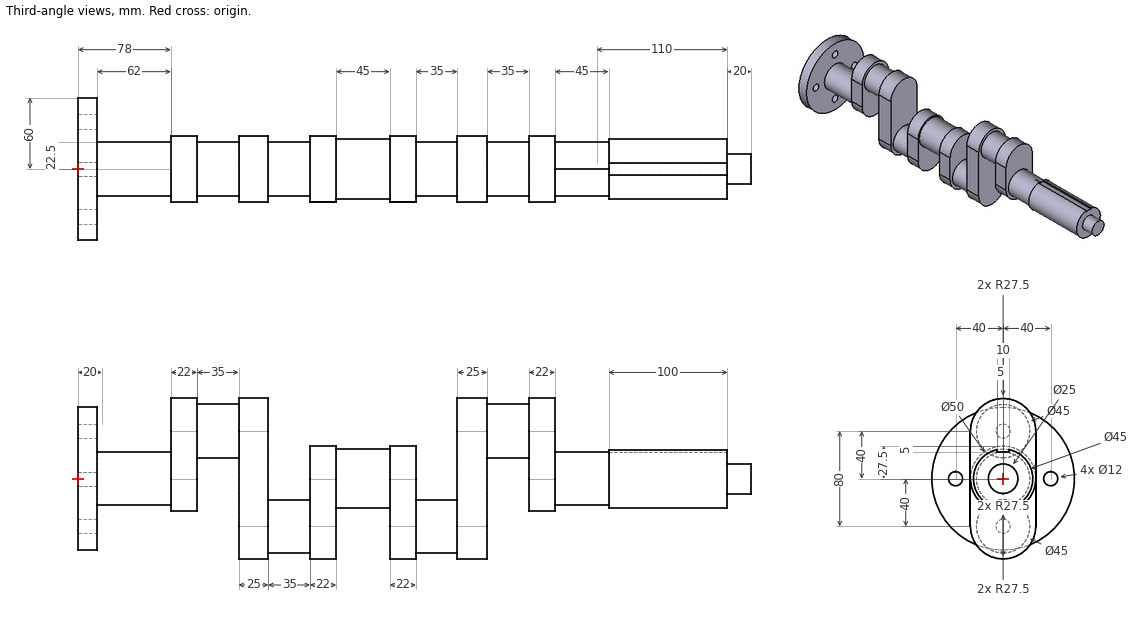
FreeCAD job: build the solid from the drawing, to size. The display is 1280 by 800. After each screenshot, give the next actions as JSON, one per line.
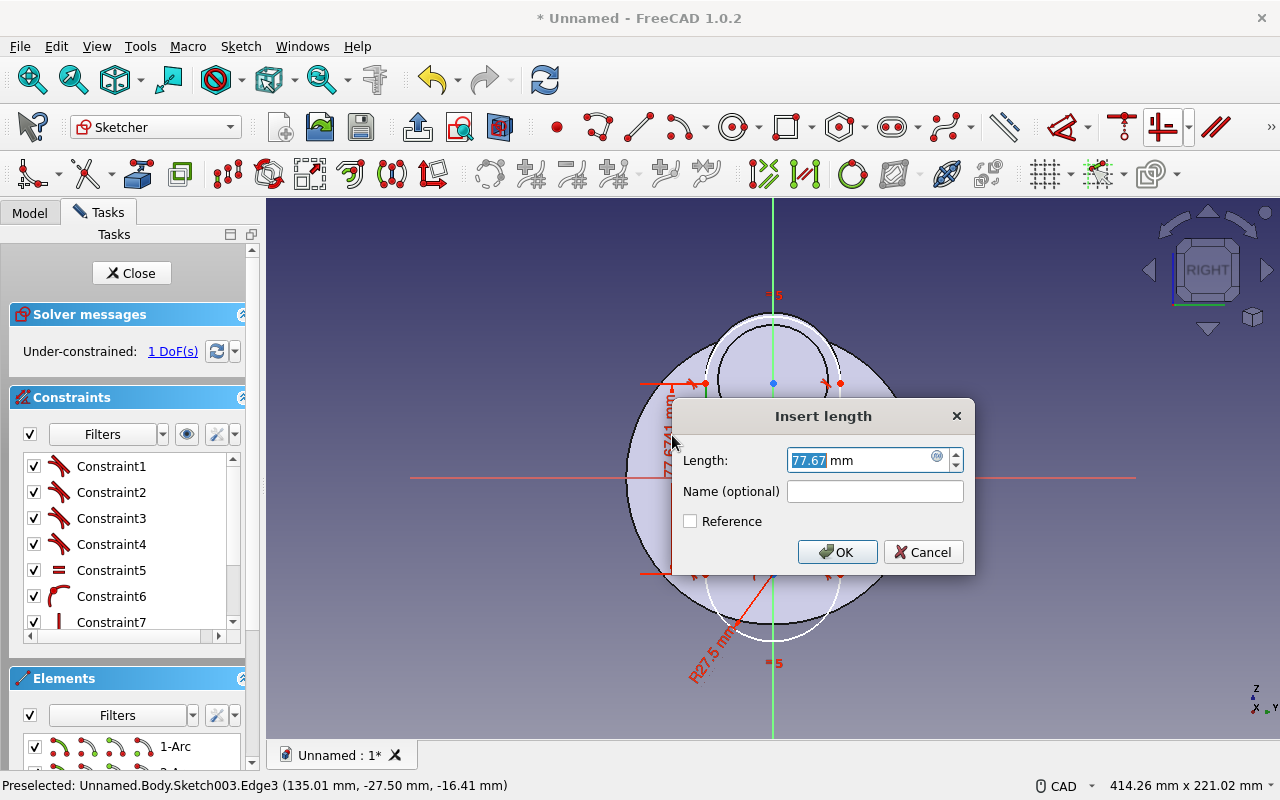
{"action": "type", "text": "80"}
{"action": "key", "text": "Return"}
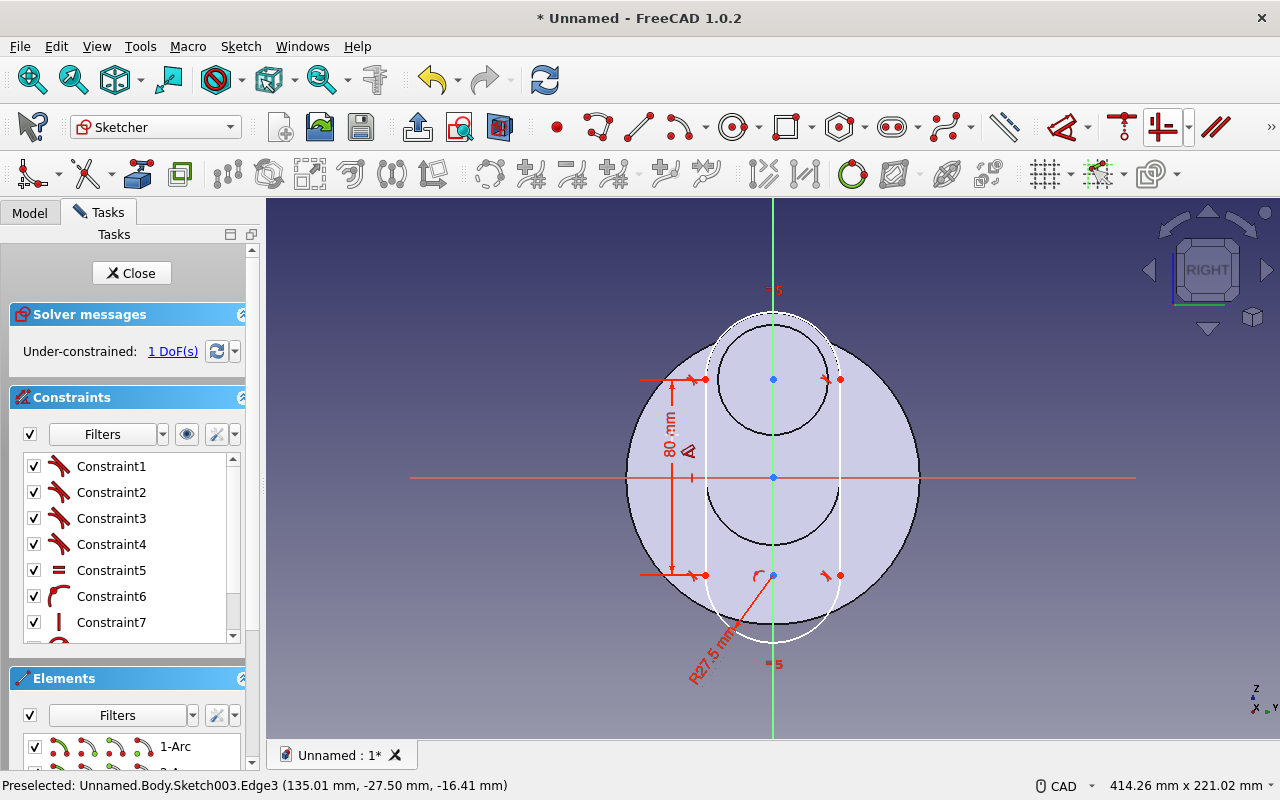
{"action": "left_click", "coordinate": [706, 575]}
{"action": "left_click", "coordinate": [672, 527]}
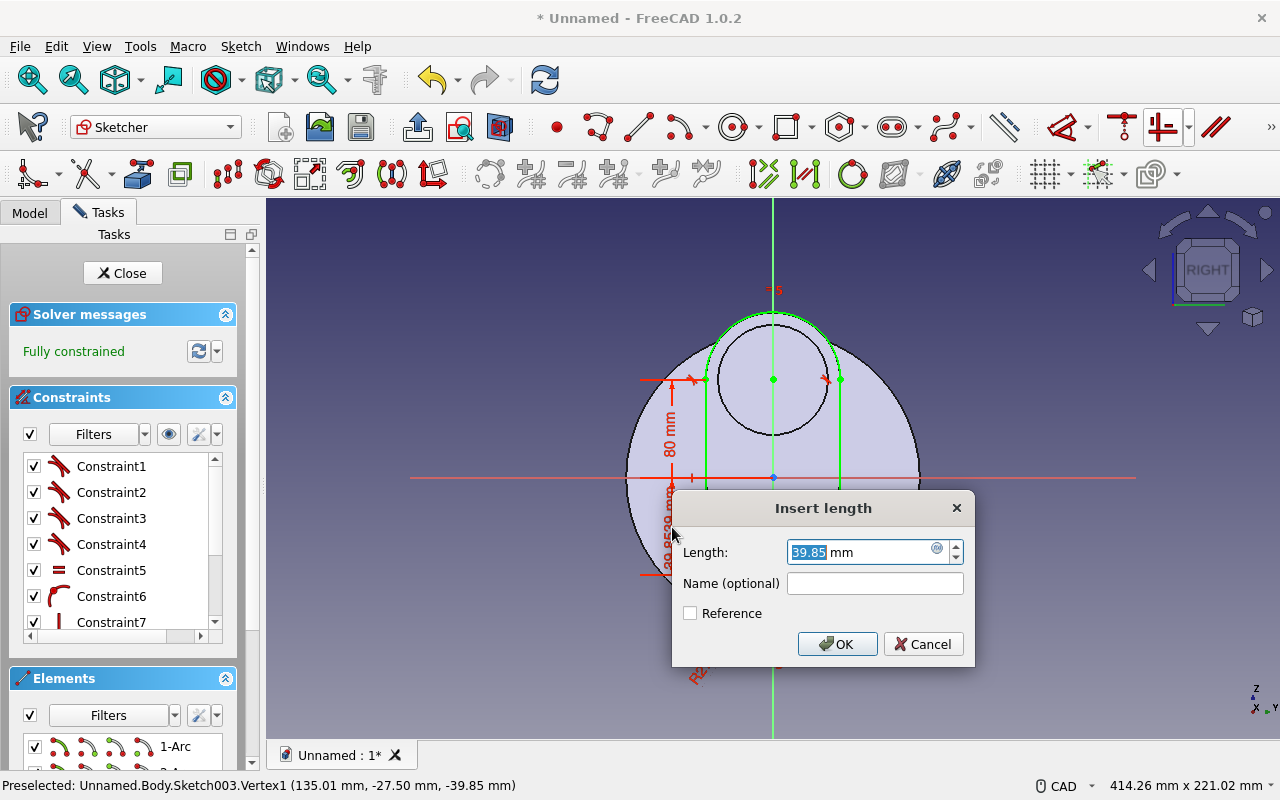
{"action": "type", "text": "40"}
{"action": "key", "text": "Return"}
{"action": "key", "text": "Escape"}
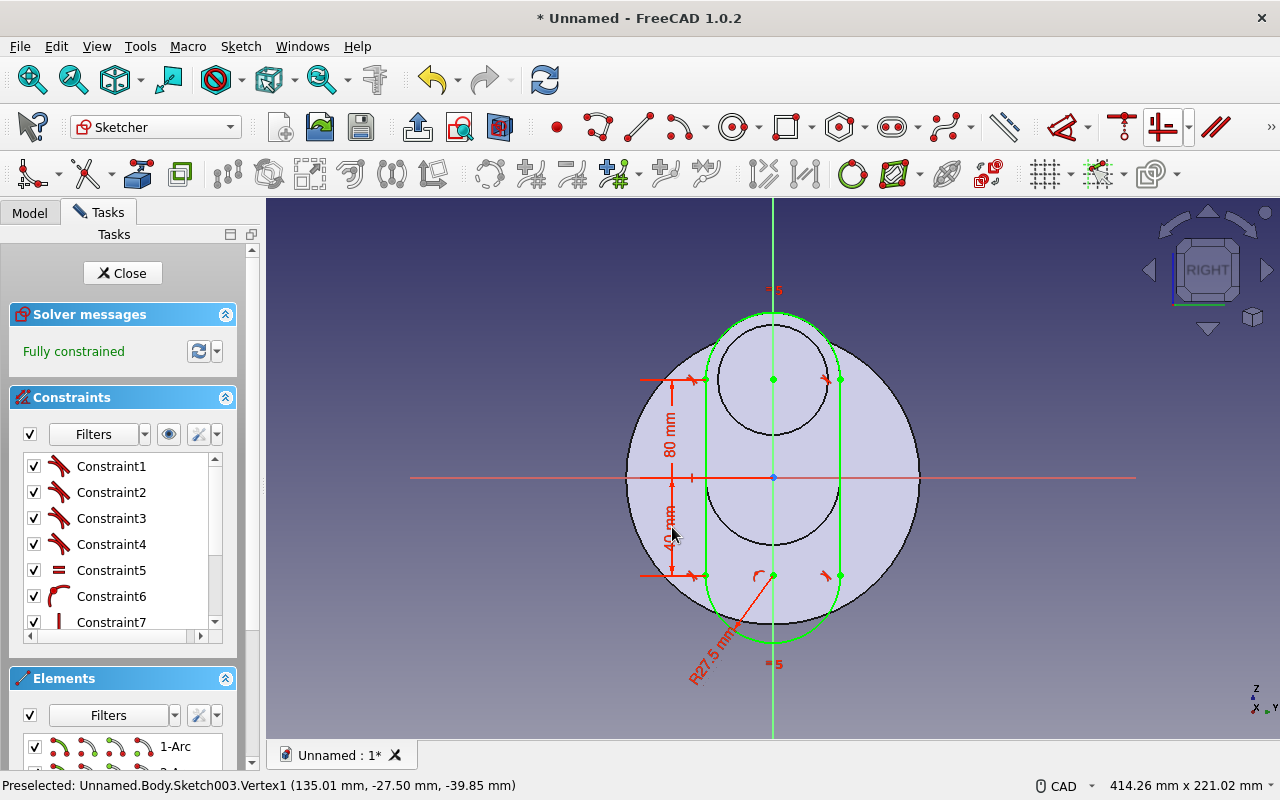
{"action": "left_click", "coordinate": [123, 273]}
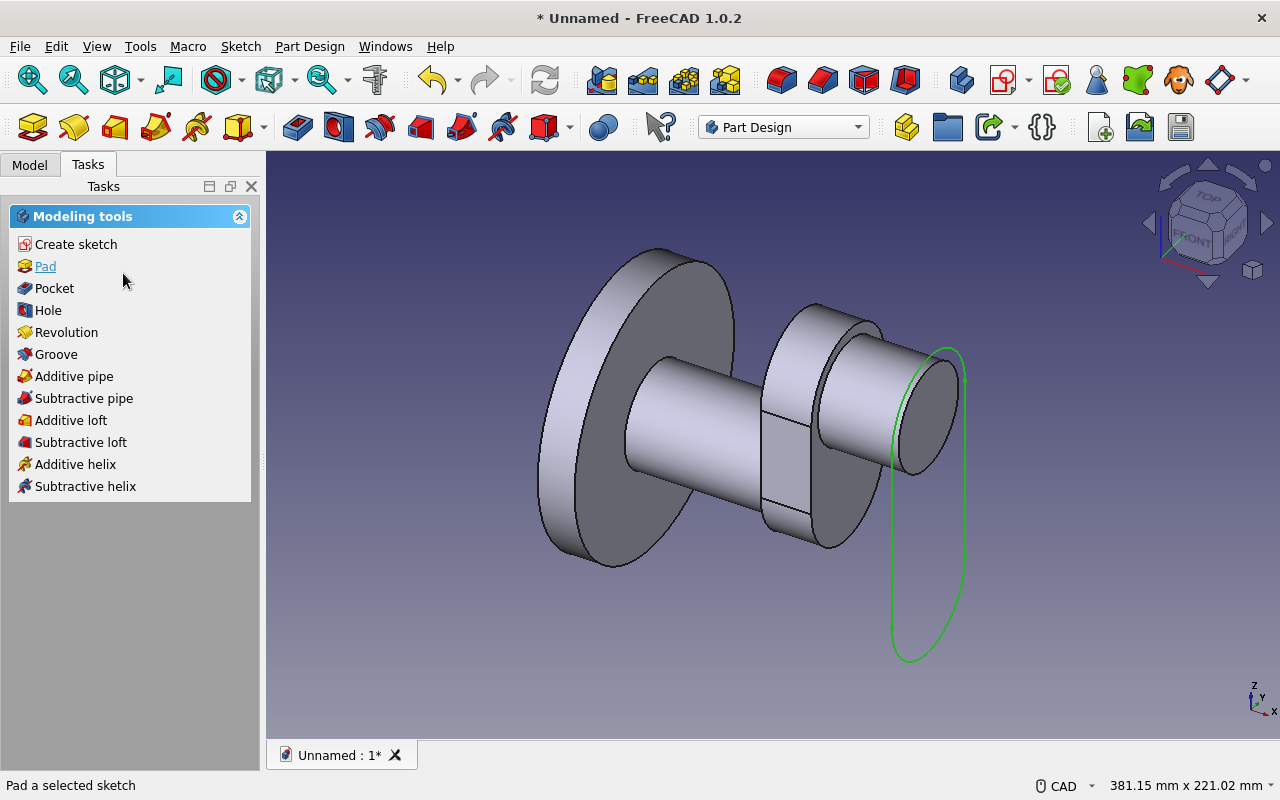
{"action": "left_click", "coordinate": [33, 128]}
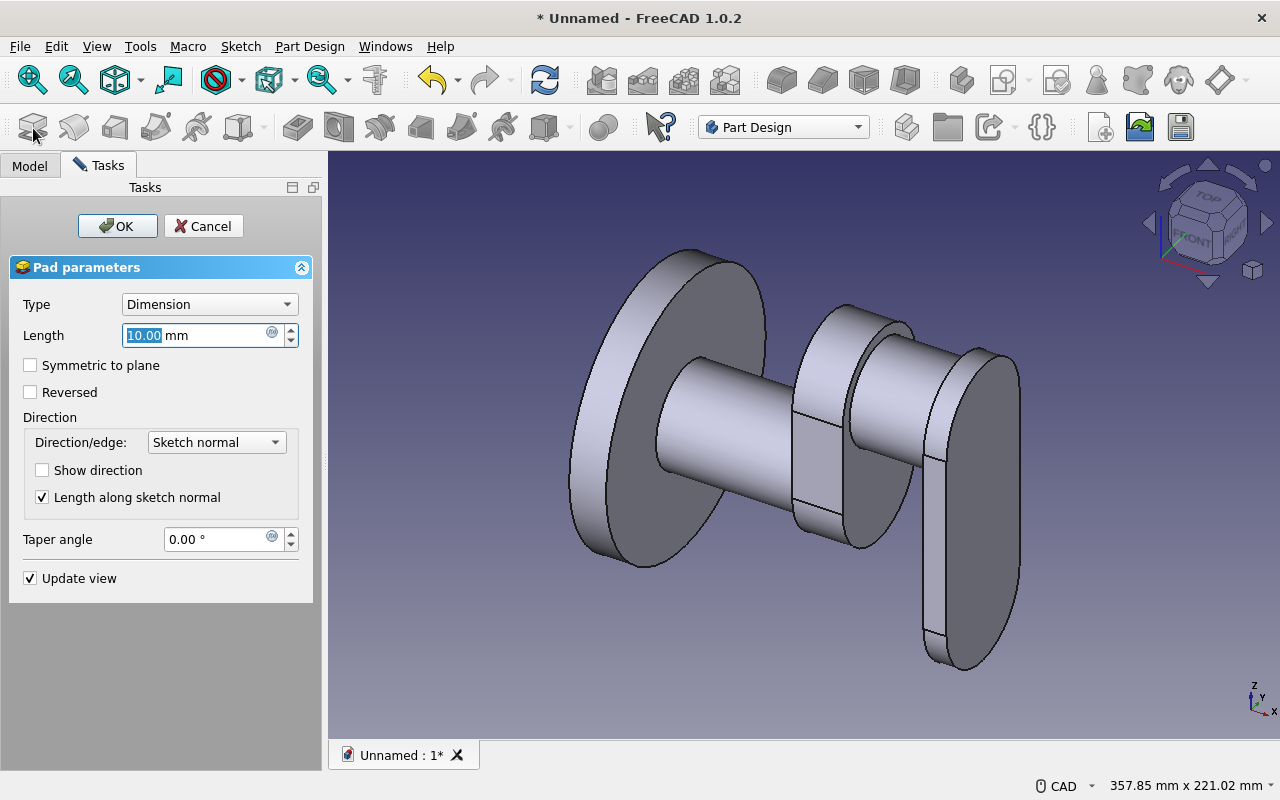
{"action": "type", "text": "25"}
{"action": "key", "text": "Tab"}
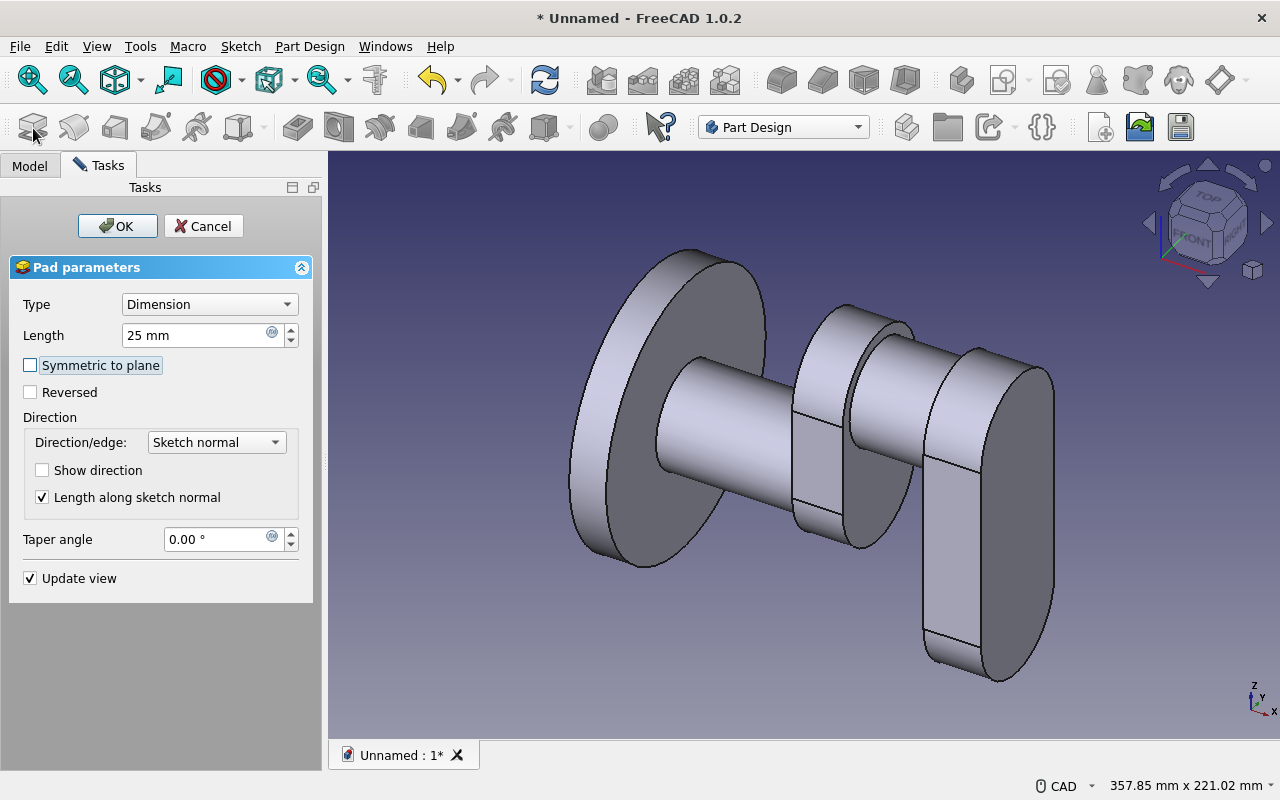
{"action": "left_click", "coordinate": [118, 226]}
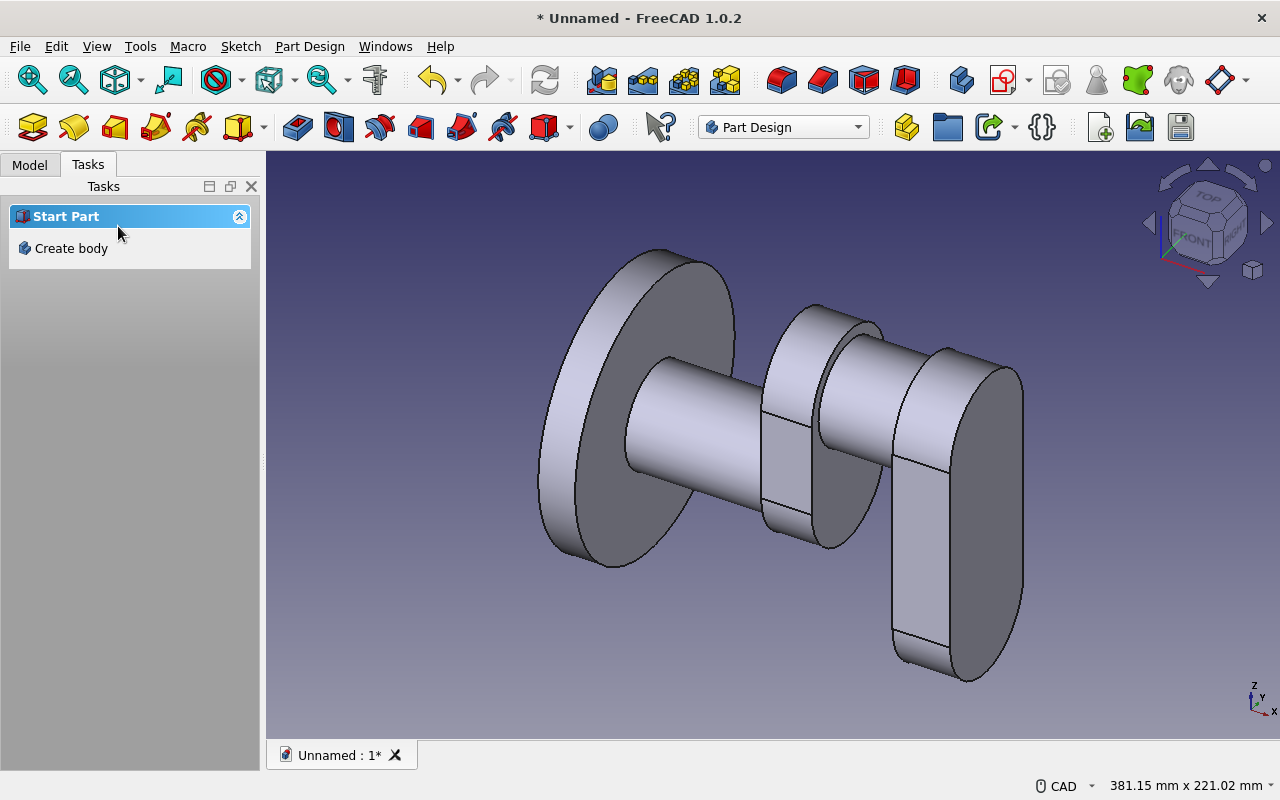
{"action": "left_click", "coordinate": [33, 80]}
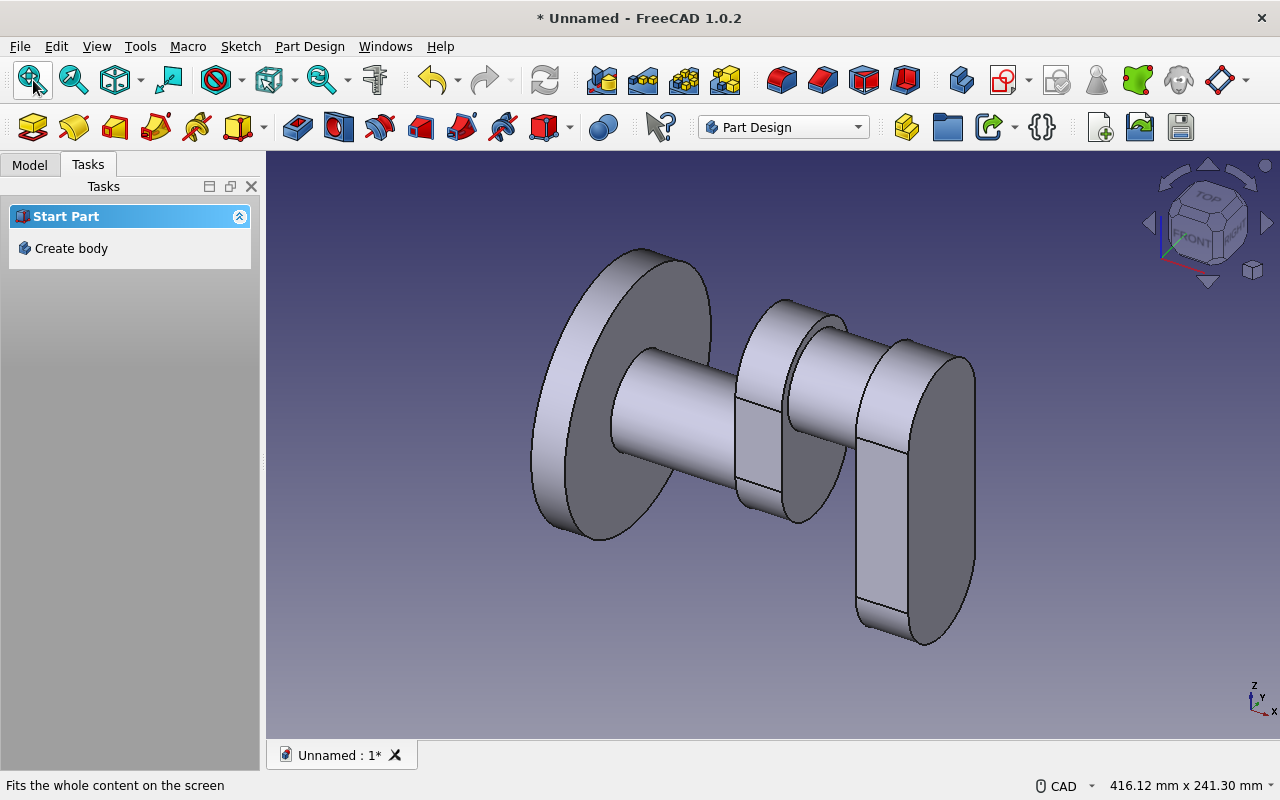
{"action": "left_click", "coordinate": [942, 423]}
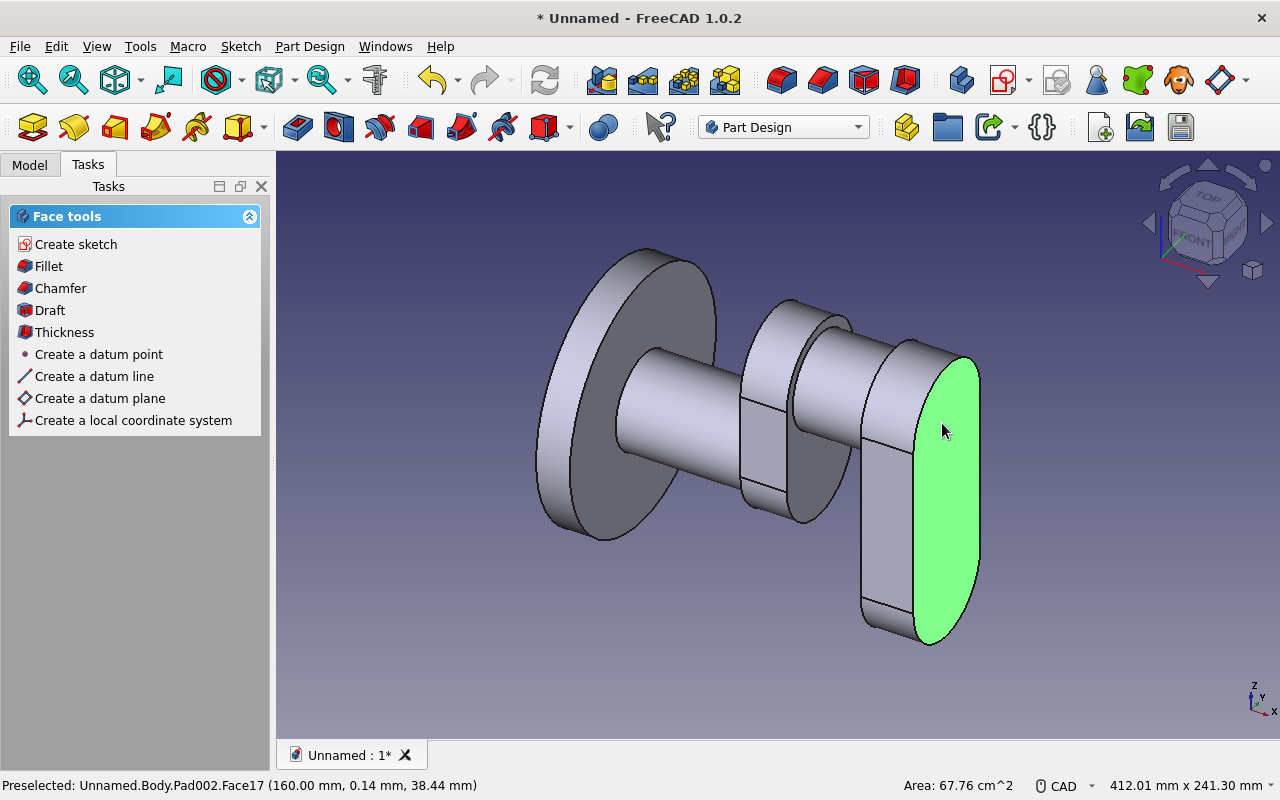
{"action": "left_click", "coordinate": [1002, 80]}